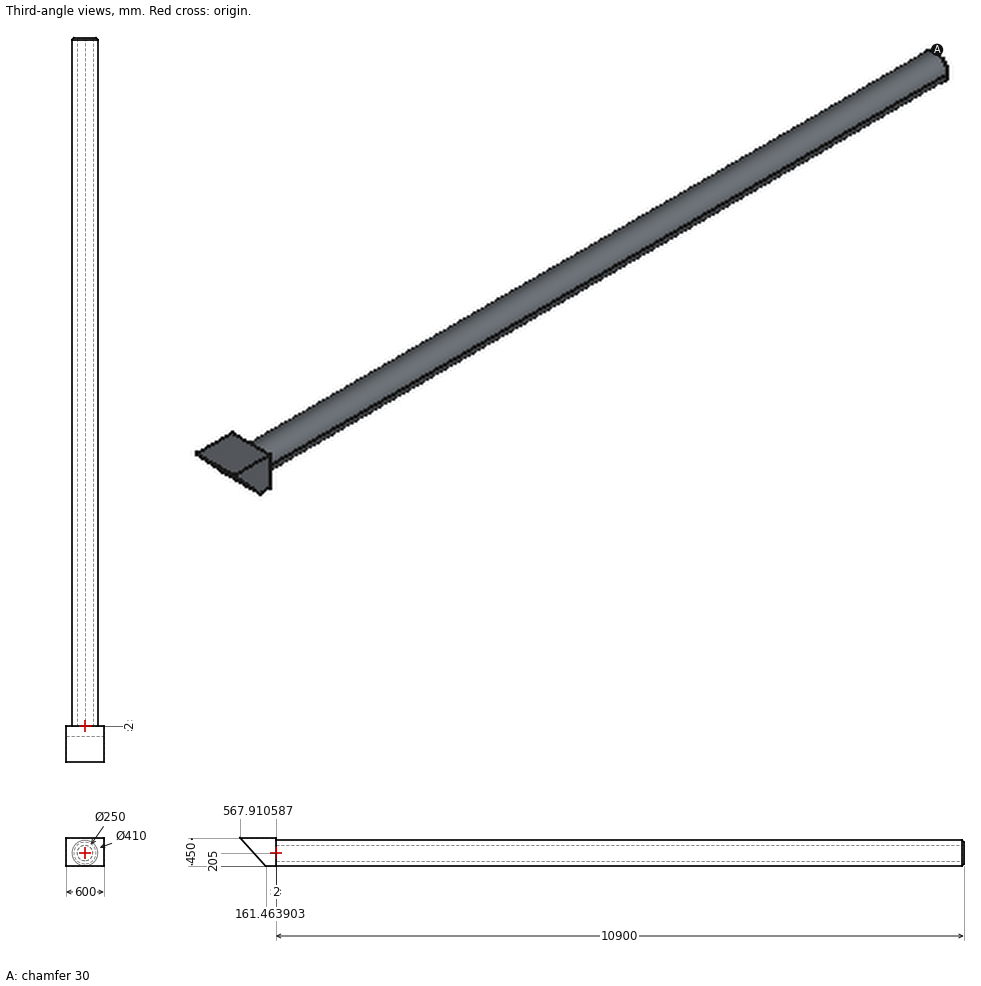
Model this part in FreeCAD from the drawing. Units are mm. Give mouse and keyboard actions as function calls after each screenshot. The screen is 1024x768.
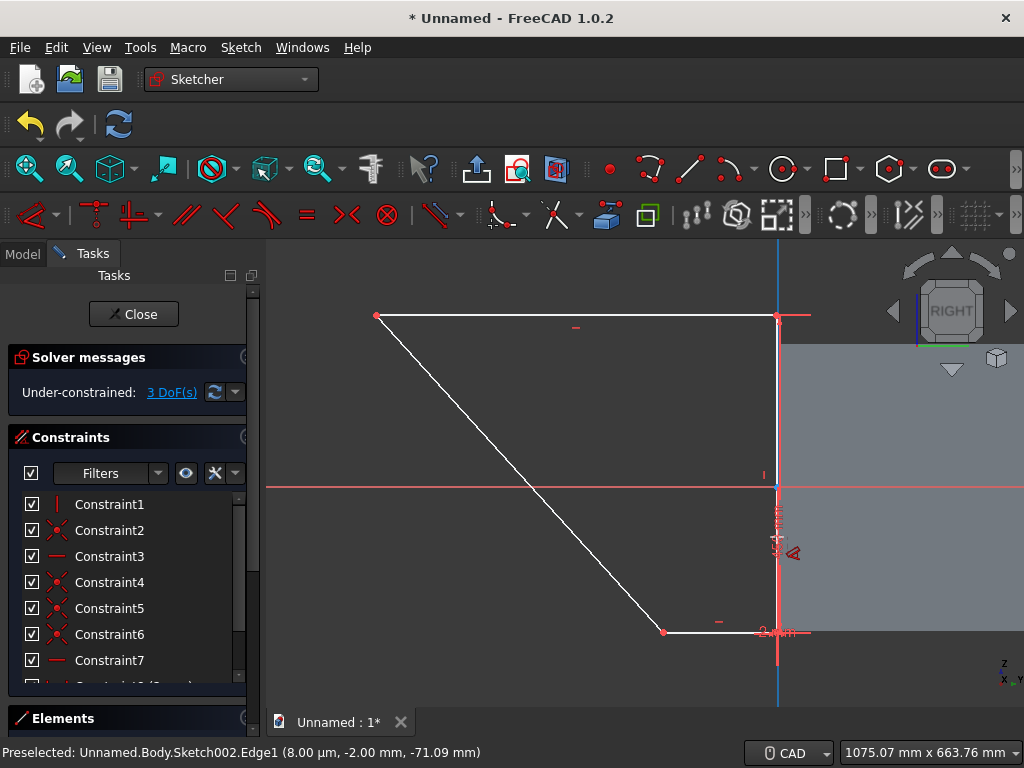
click(777, 633)
click(812, 560)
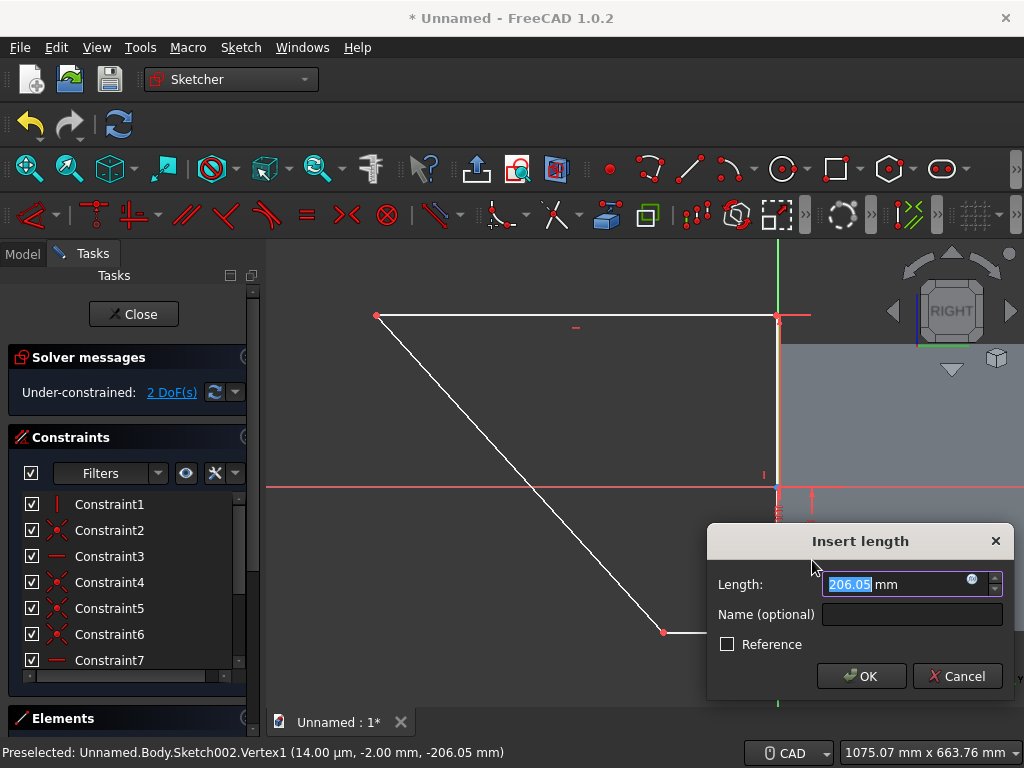
text(205)
key(Return)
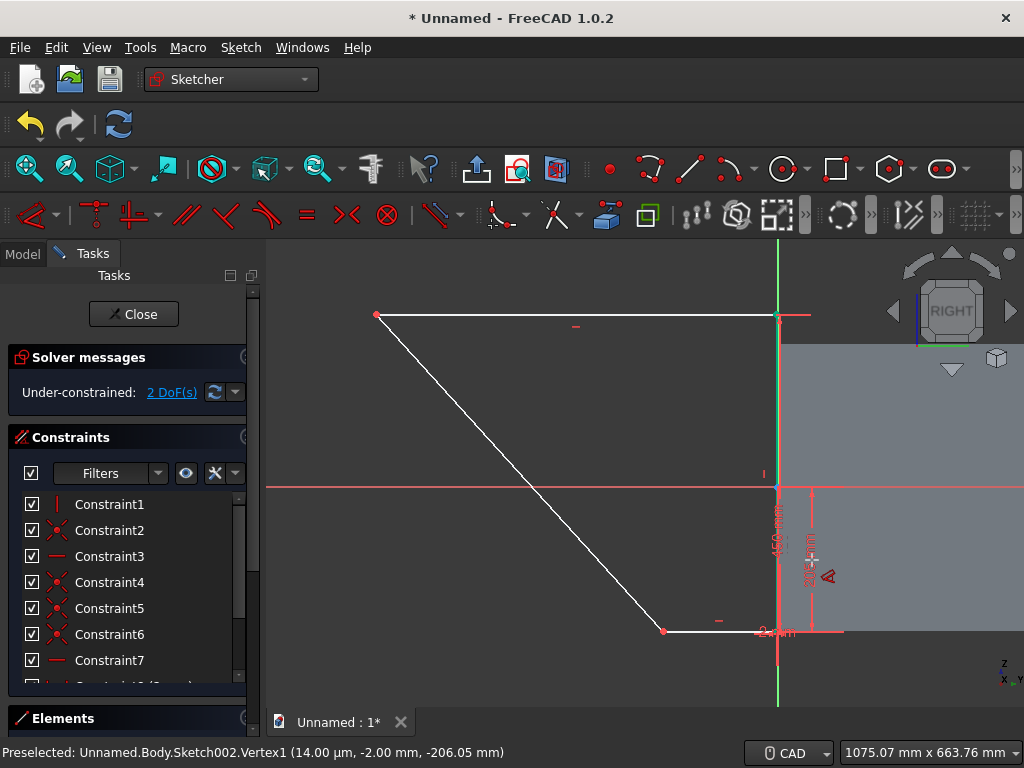
click(656, 315)
click(576, 281)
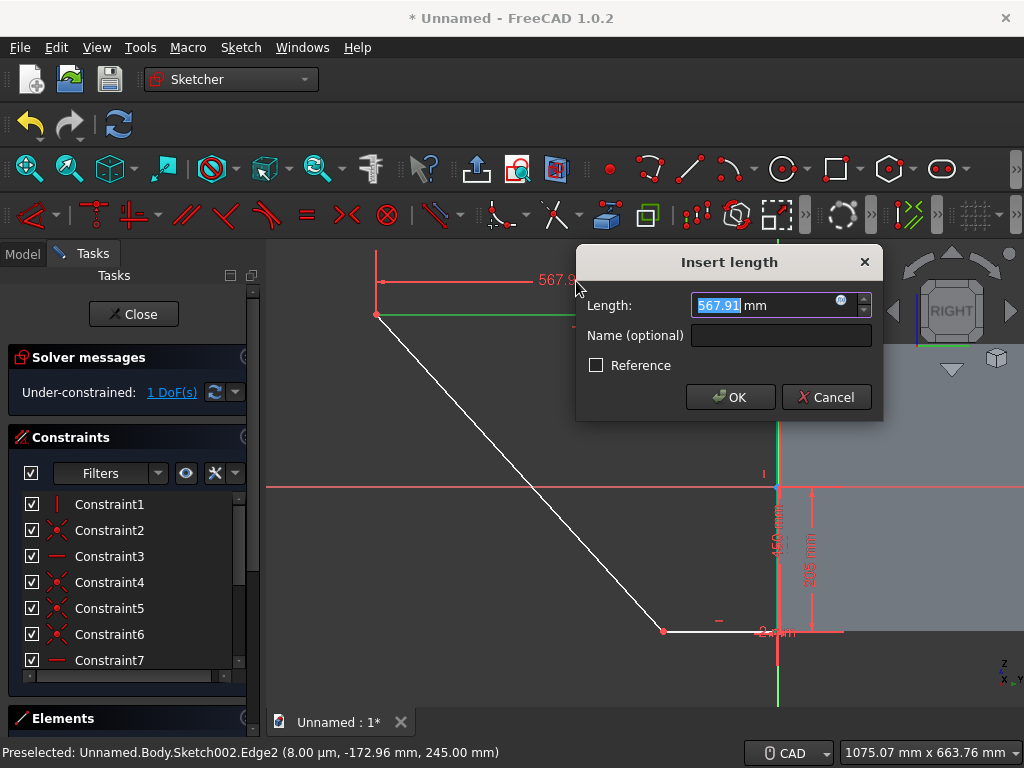
text(567.910587)
key(Return)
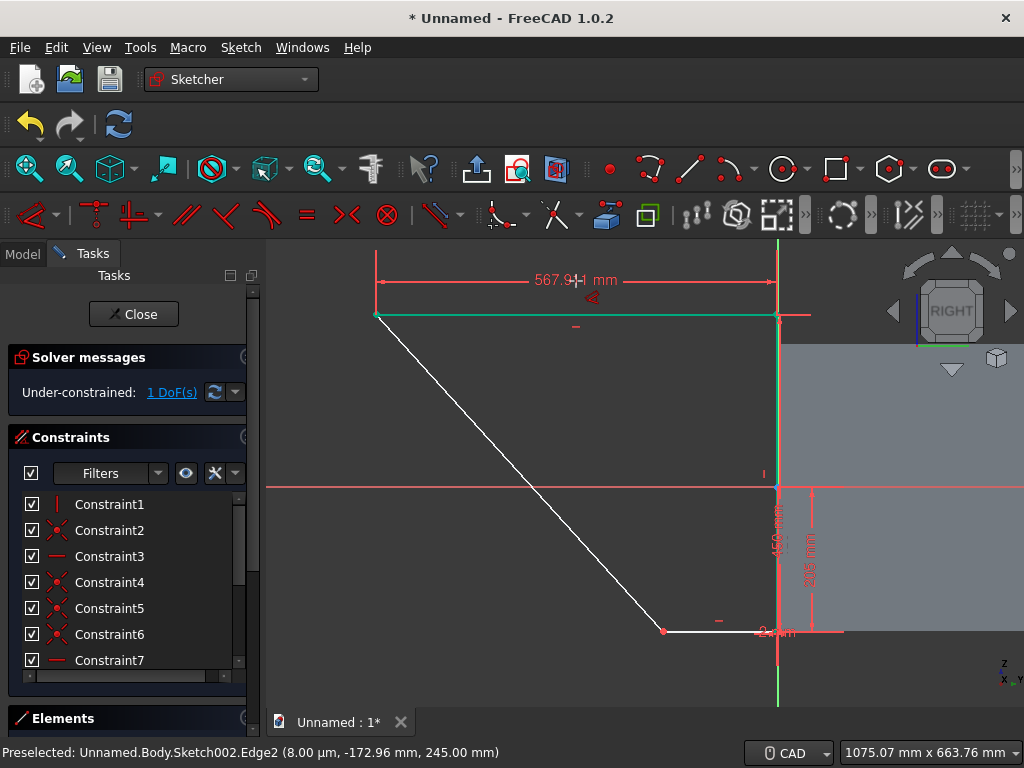
click(697, 632)
click(720, 666)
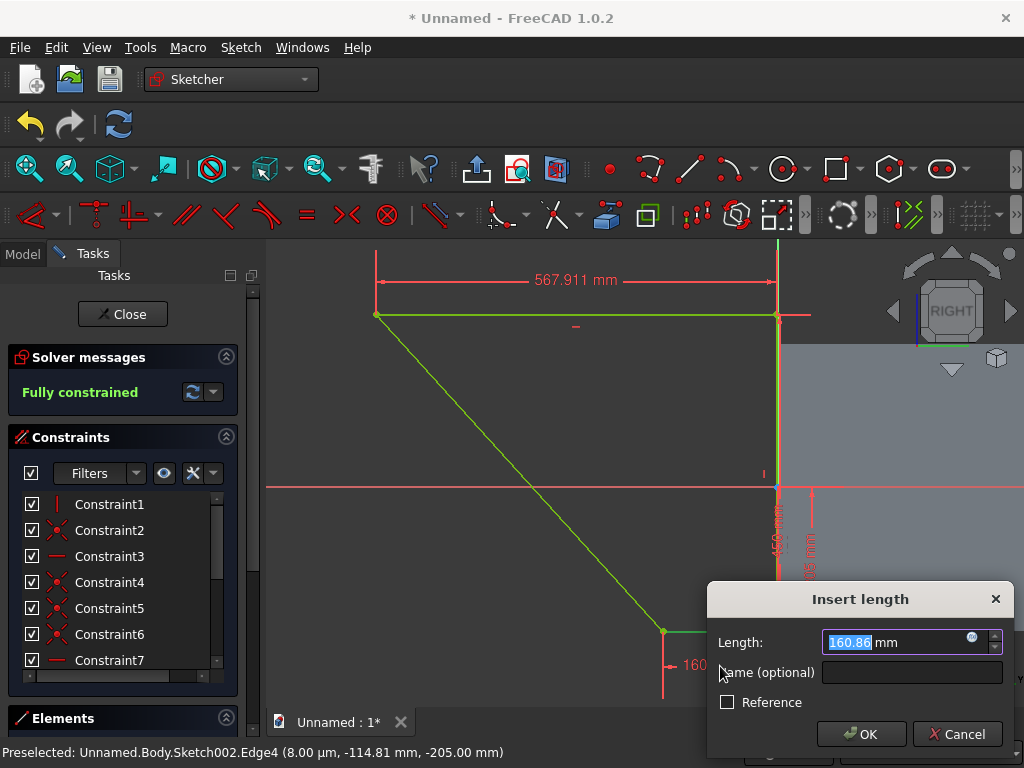
text(161.463903)
key(Return)
key(Escape)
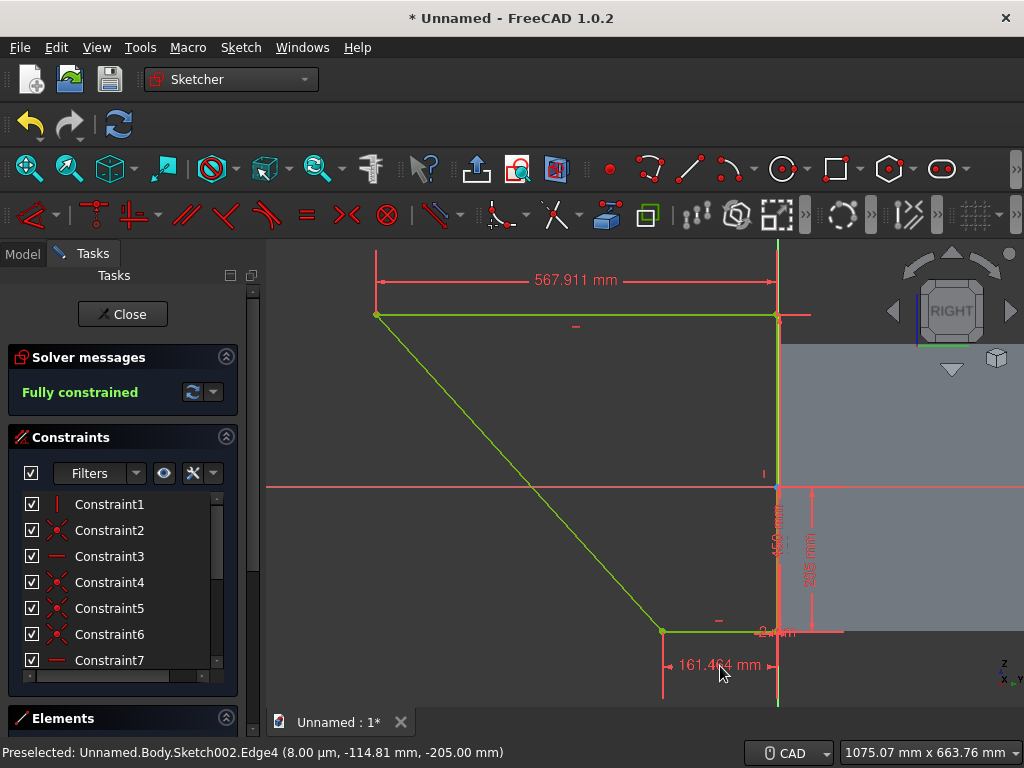
click(123, 314)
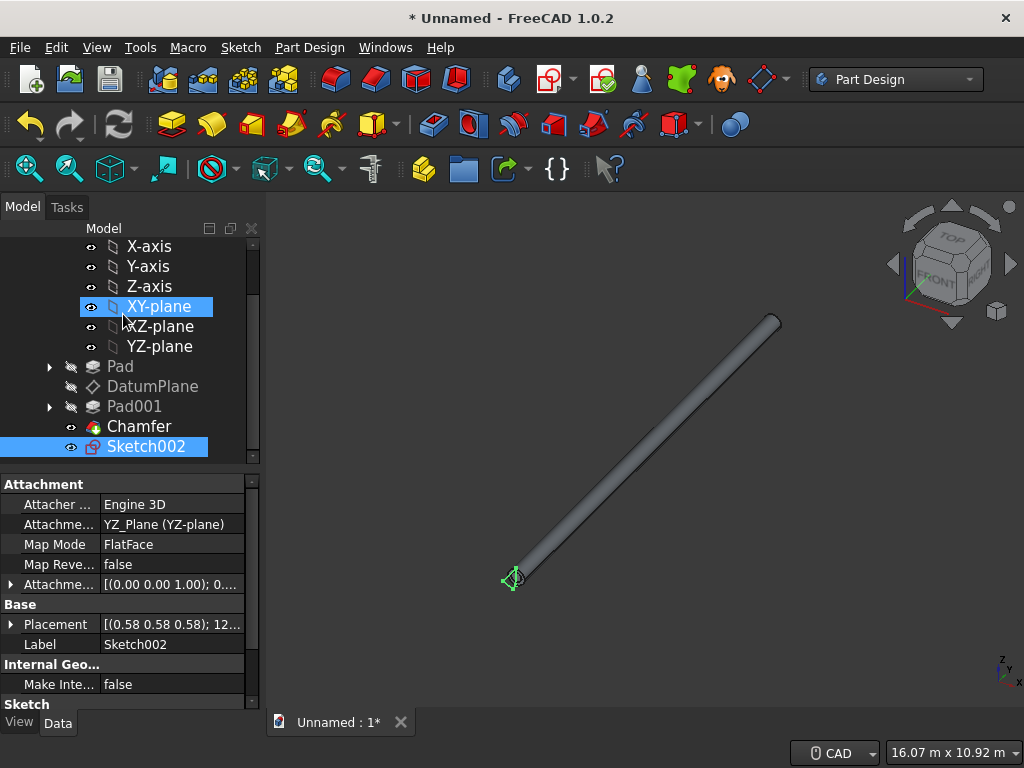
click(172, 124)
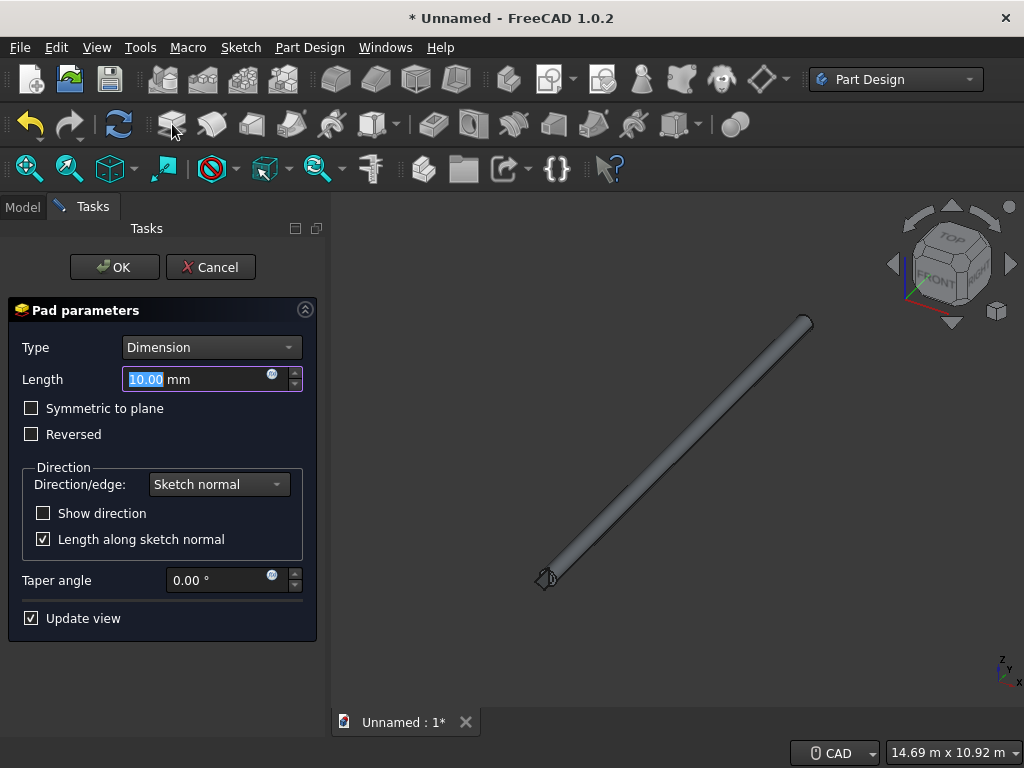
text(600)
key(Tab)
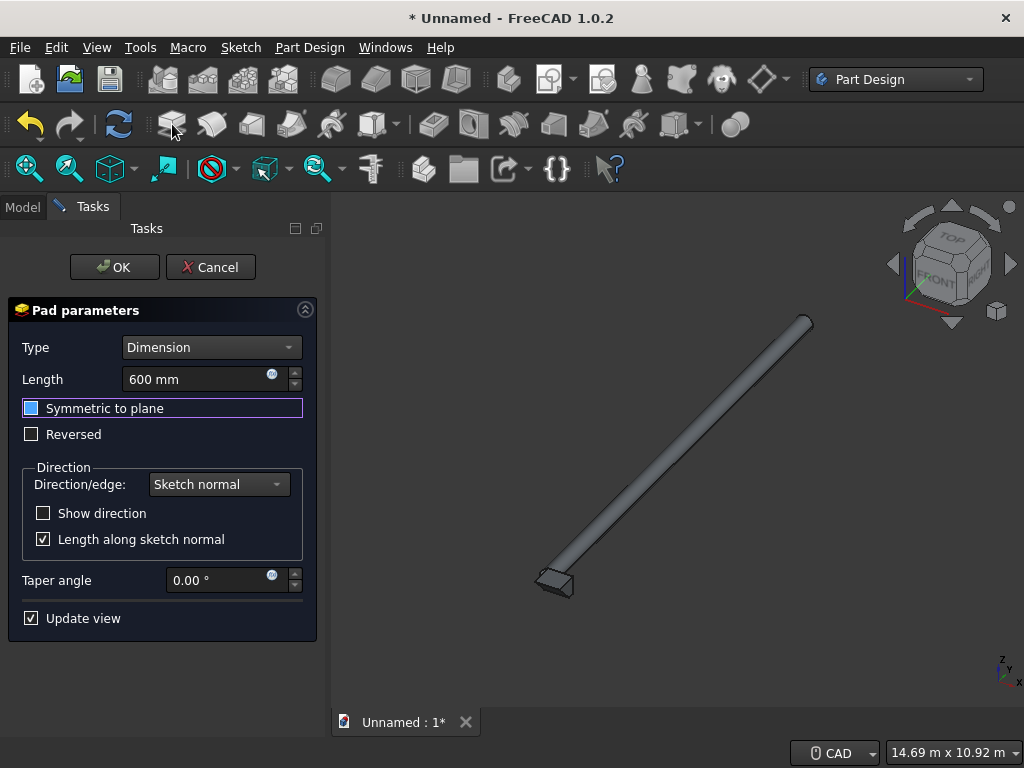
click(30, 408)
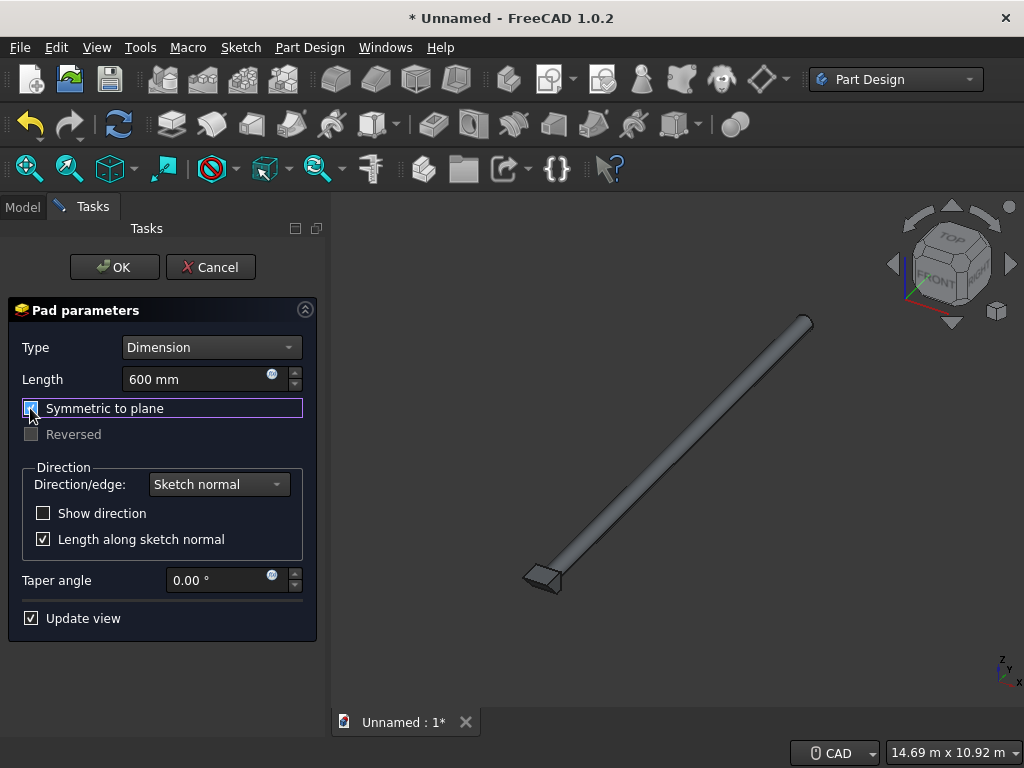
click(115, 267)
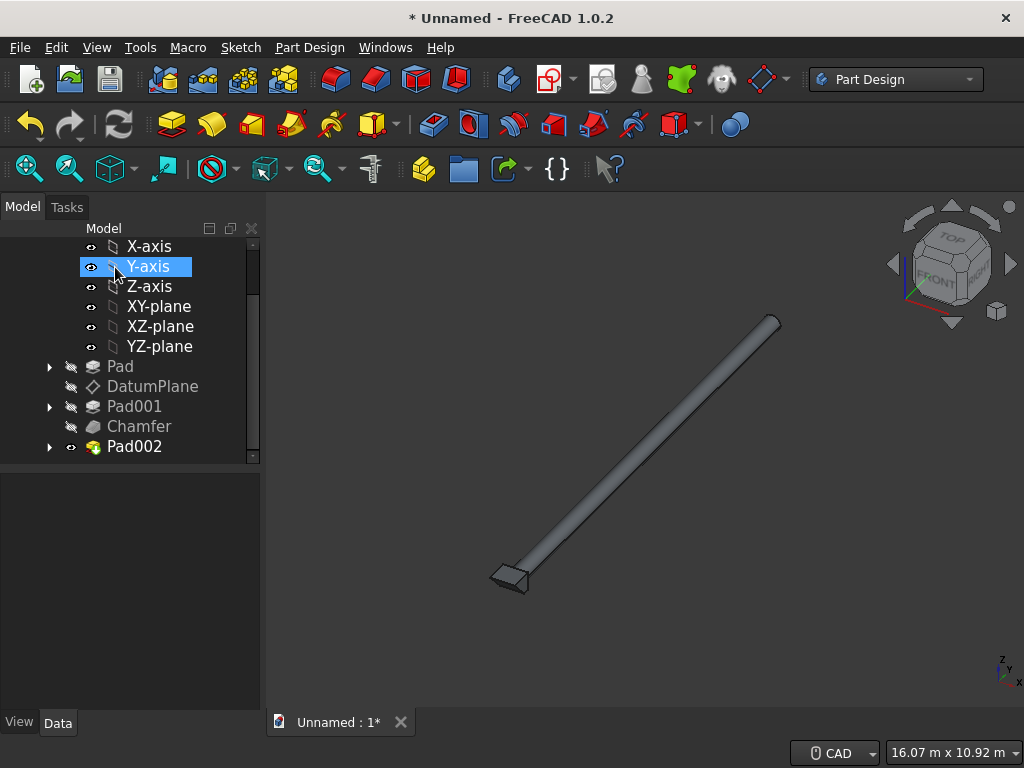
key(0)